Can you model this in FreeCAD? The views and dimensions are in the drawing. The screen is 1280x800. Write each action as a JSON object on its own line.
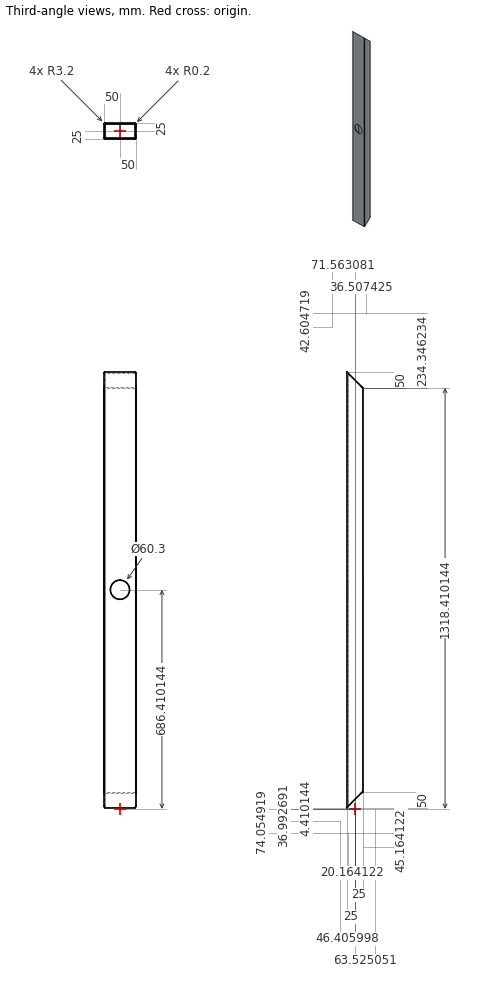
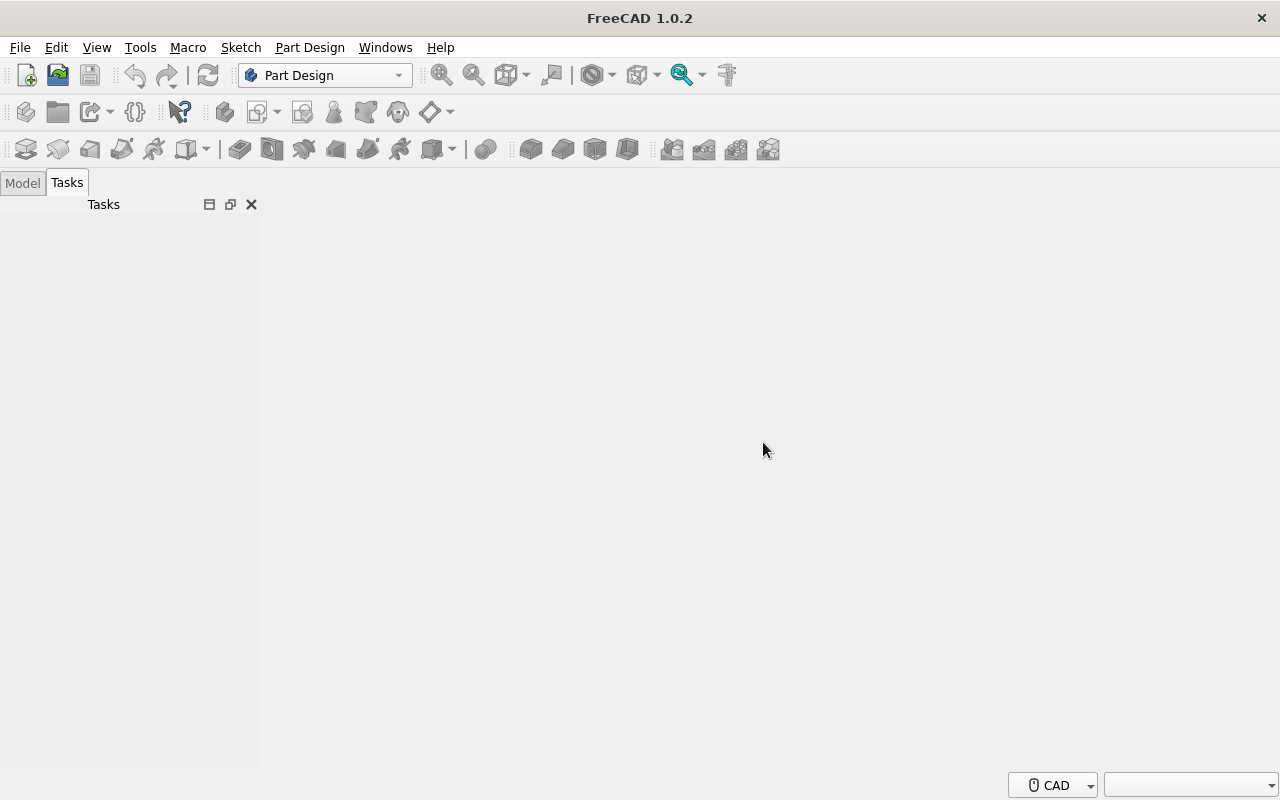
{"action": "left_click", "coordinate": [26, 76]}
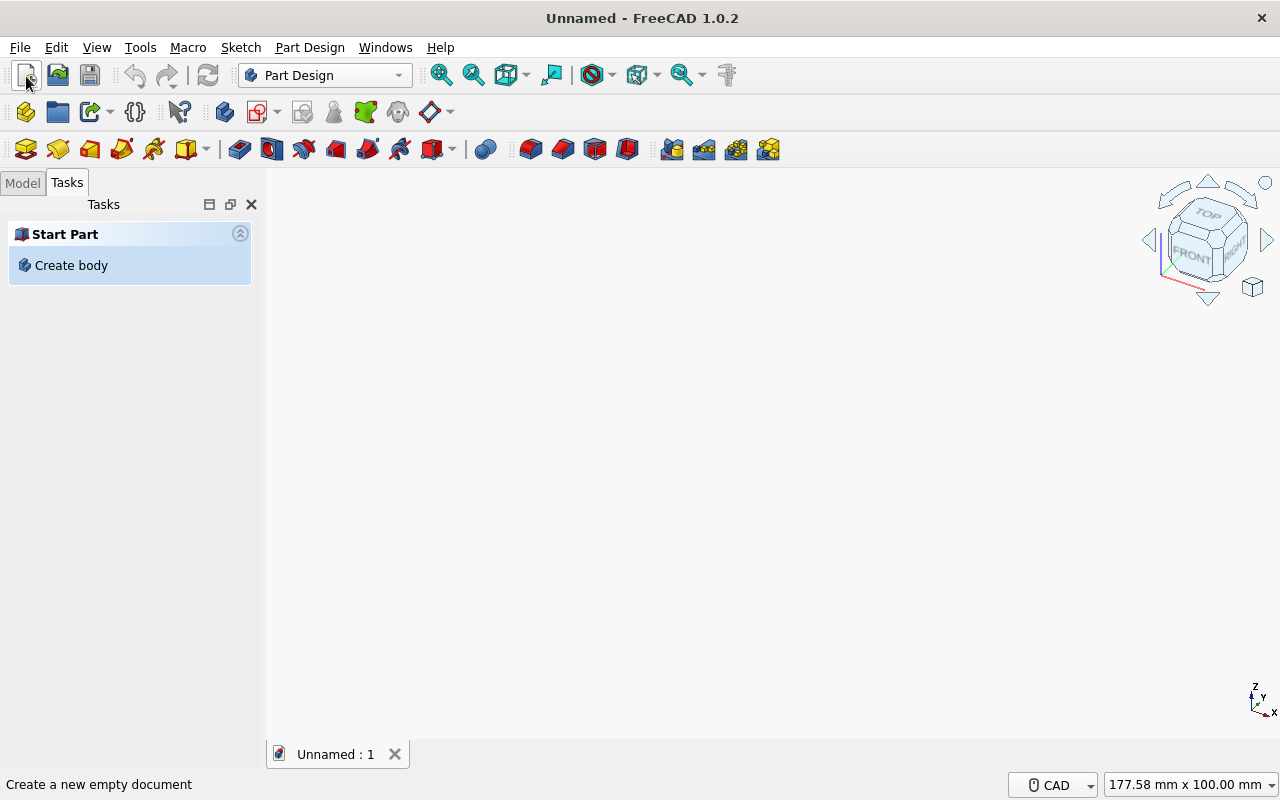
{"action": "left_click", "coordinate": [258, 112]}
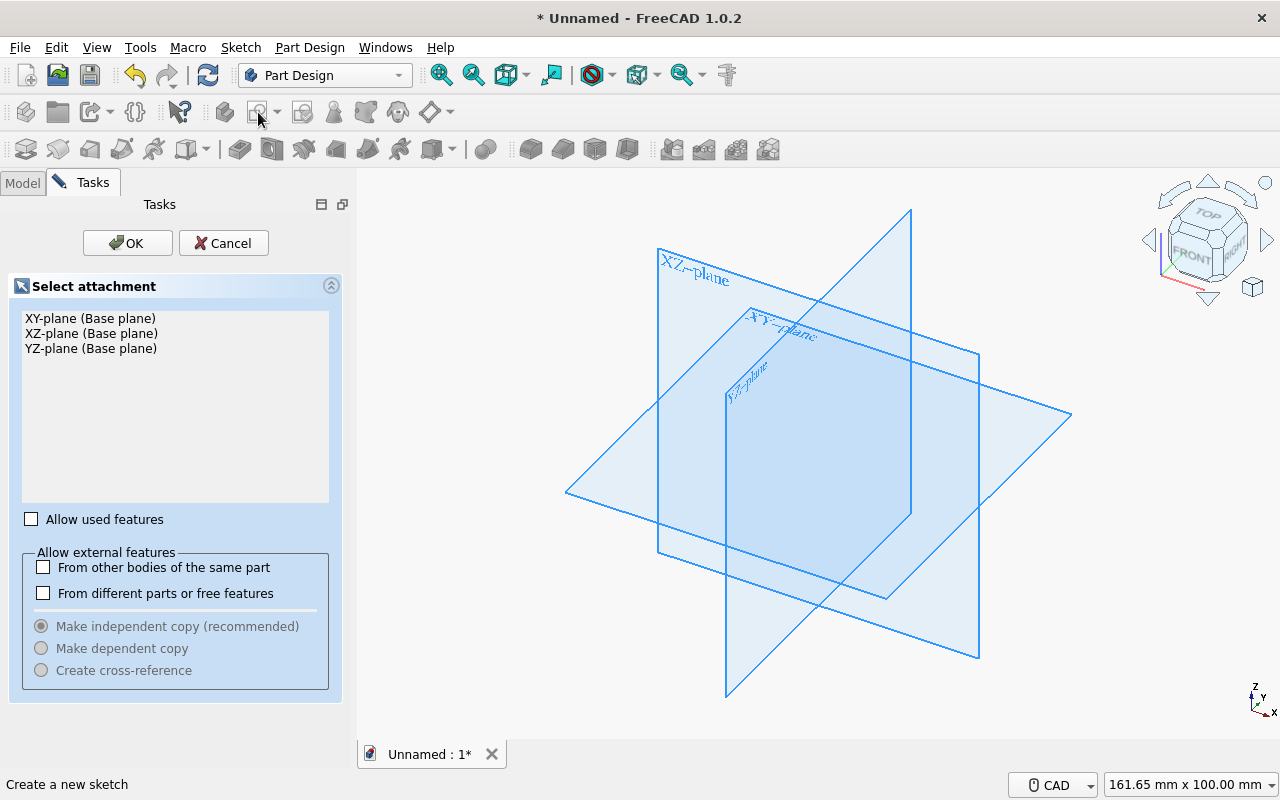
{"action": "left_click", "coordinate": [82, 318]}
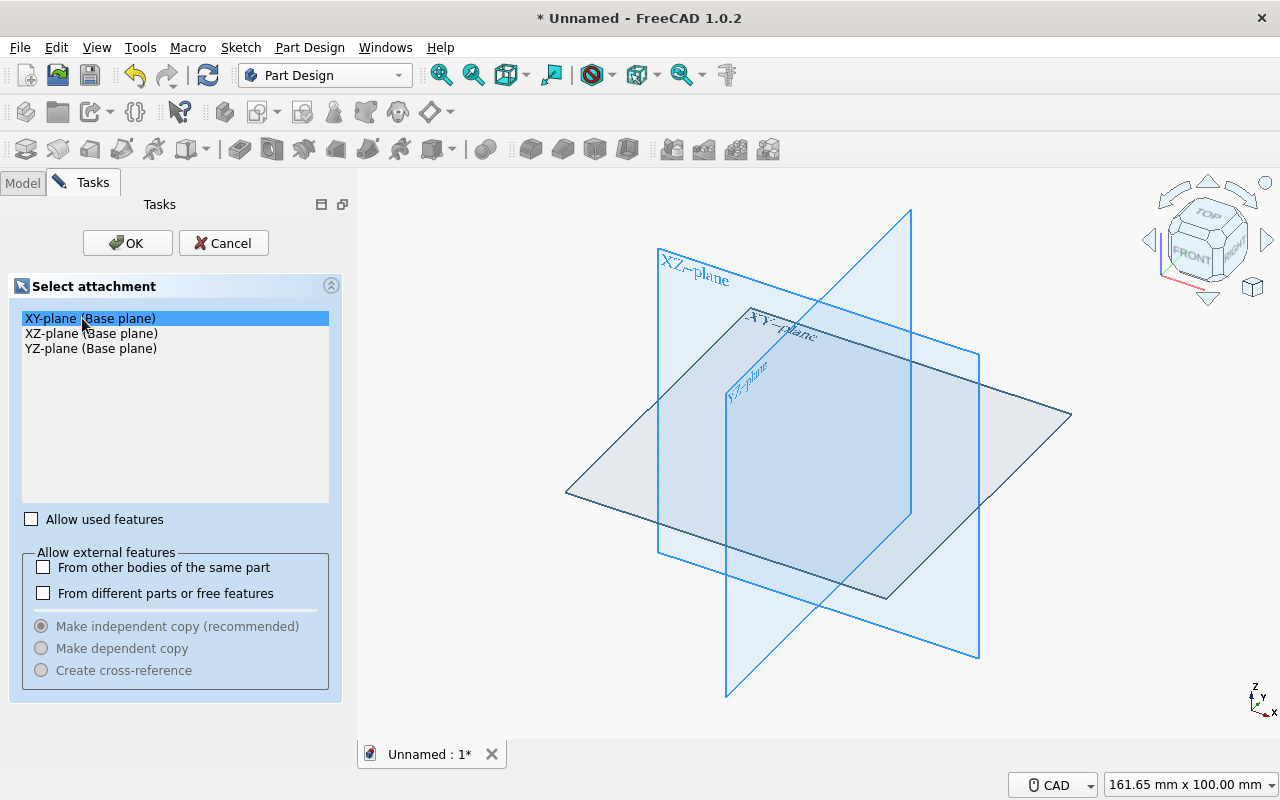
{"action": "left_click", "coordinate": [128, 243]}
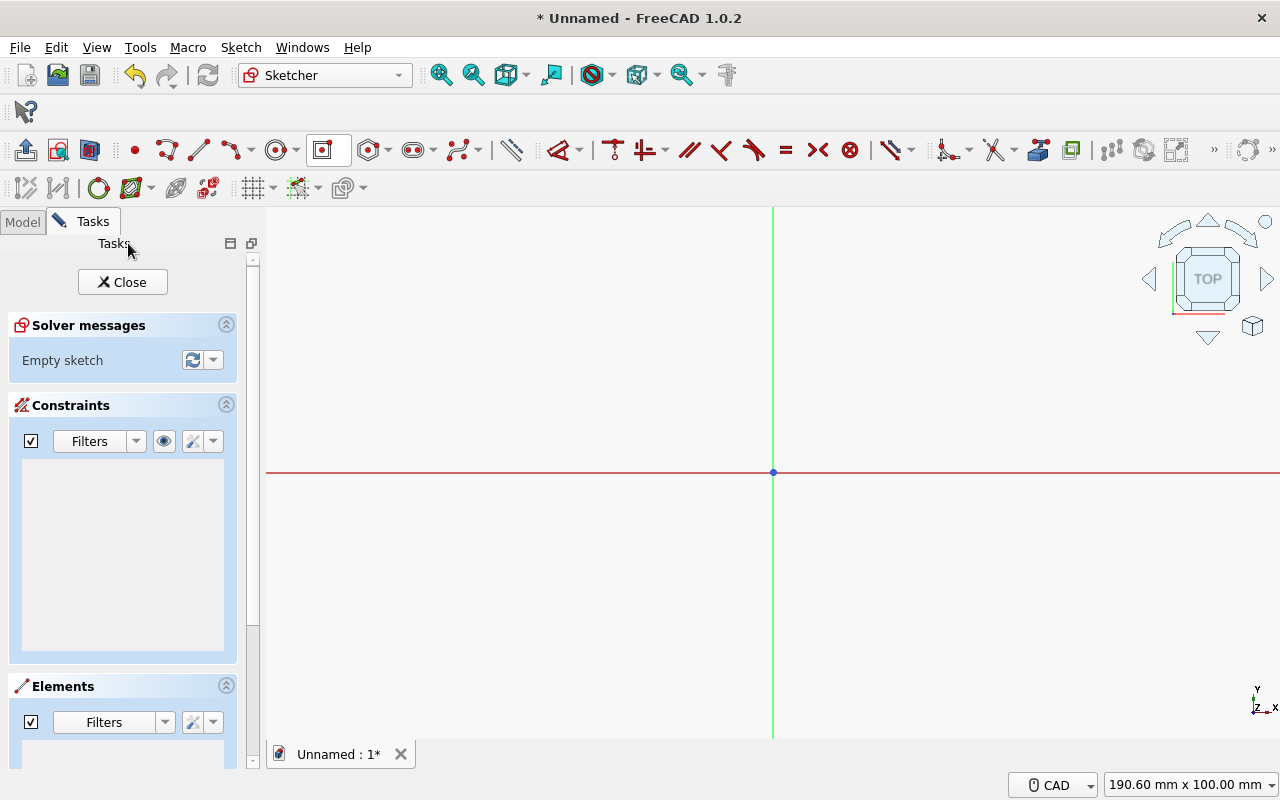
{"action": "left_click", "coordinate": [200, 150]}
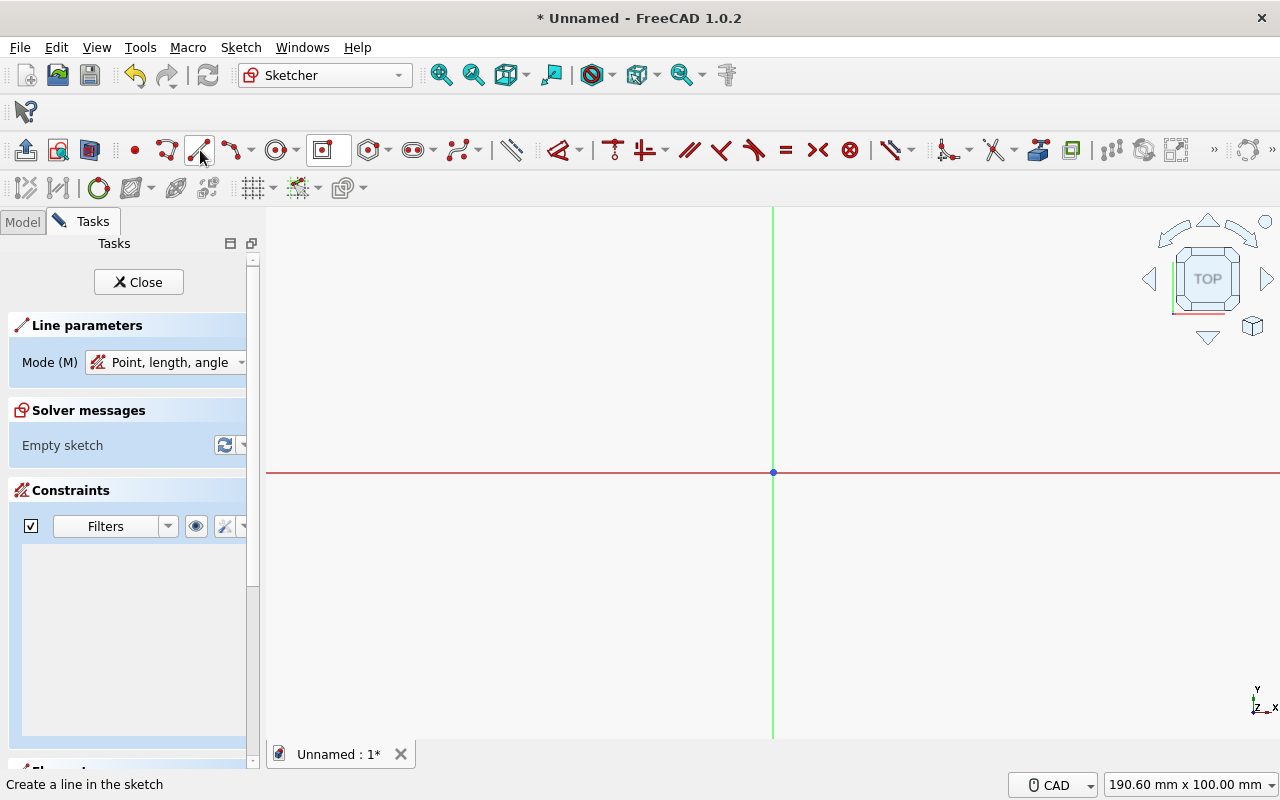
{"action": "left_click", "coordinate": [1022, 340]}
{"action": "left_click", "coordinate": [524, 340]}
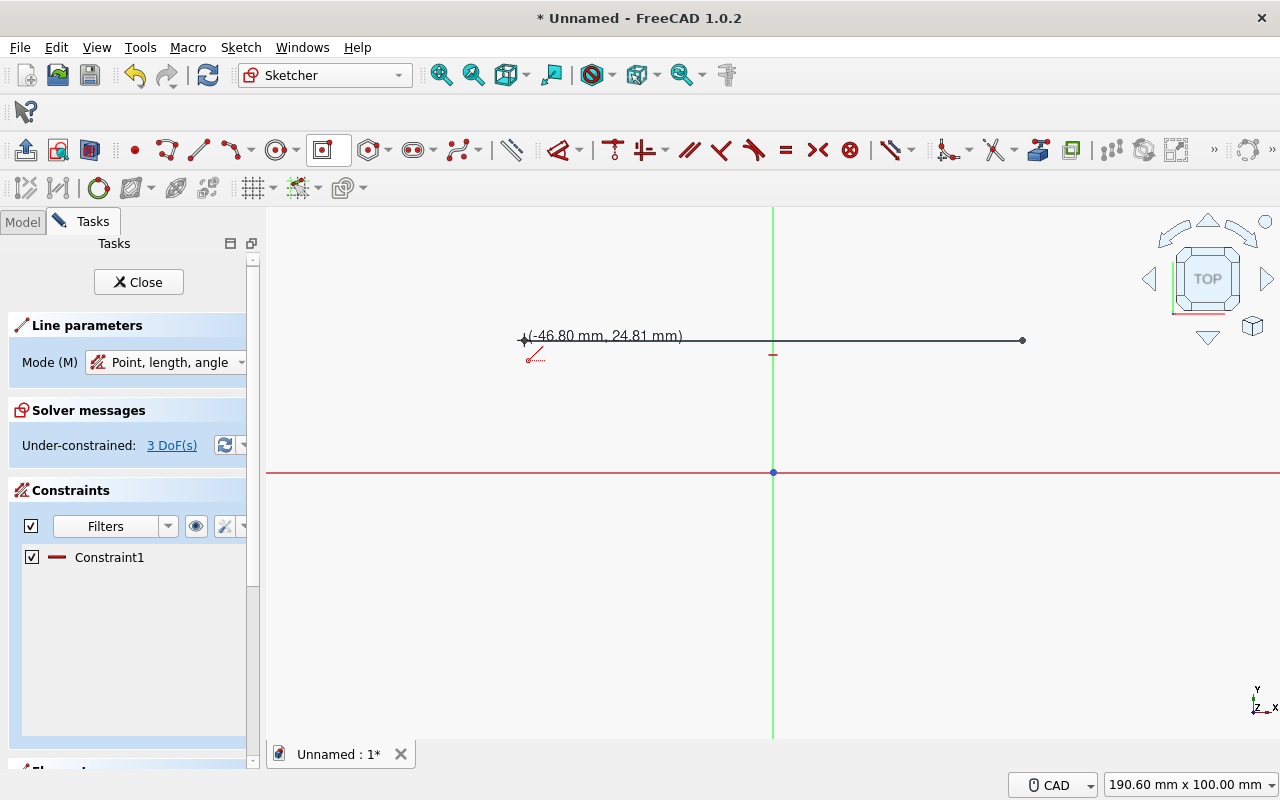
{"action": "left_click", "coordinate": [507, 357]}
{"action": "left_click", "coordinate": [507, 589]}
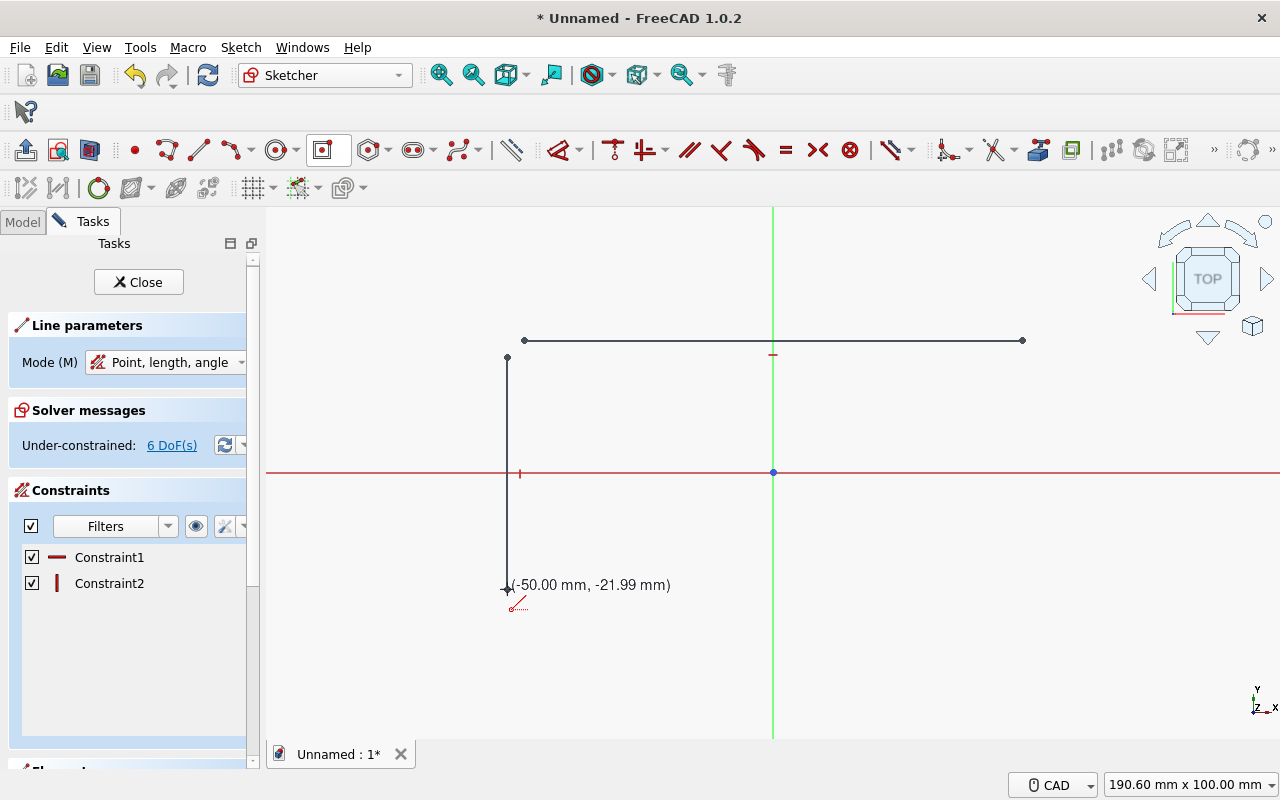
{"action": "left_click", "coordinate": [524, 606]}
{"action": "left_click", "coordinate": [1022, 606]}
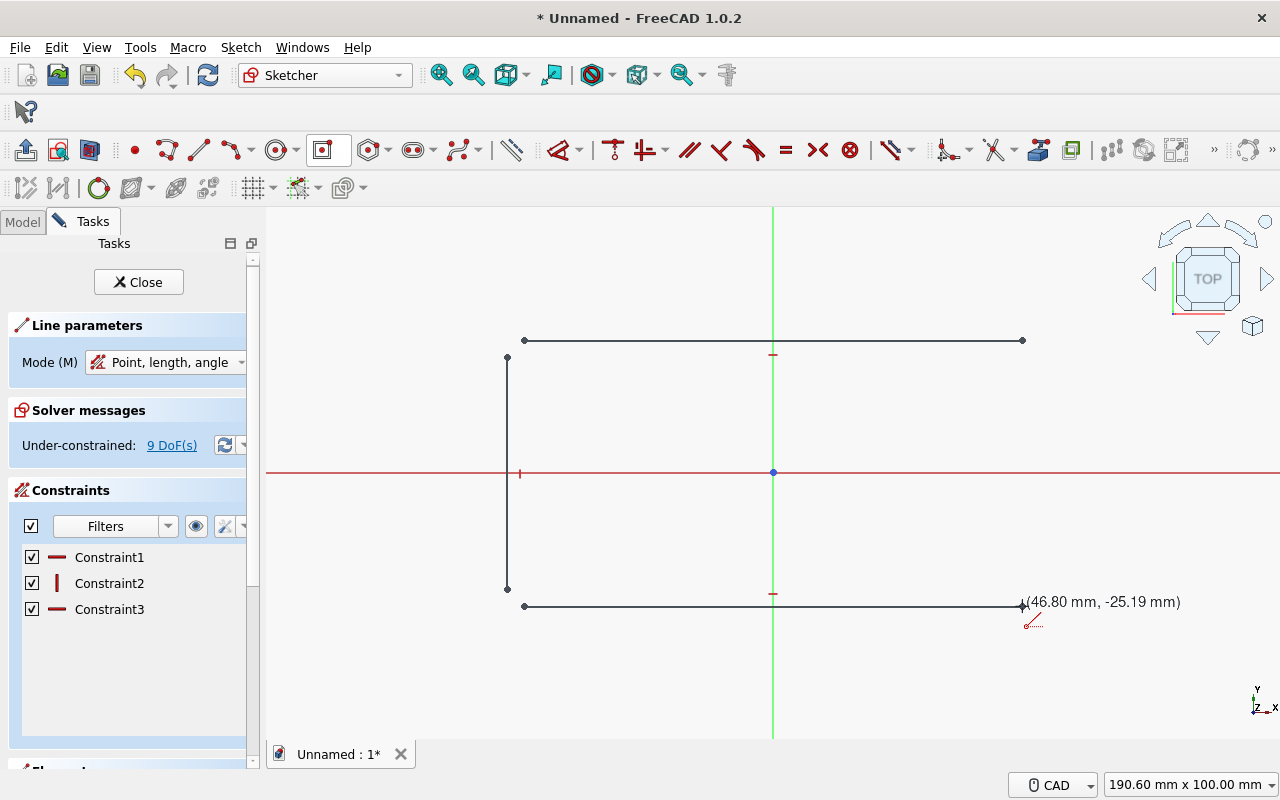
{"action": "left_click", "coordinate": [1039, 589]}
{"action": "left_click", "coordinate": [1039, 357]}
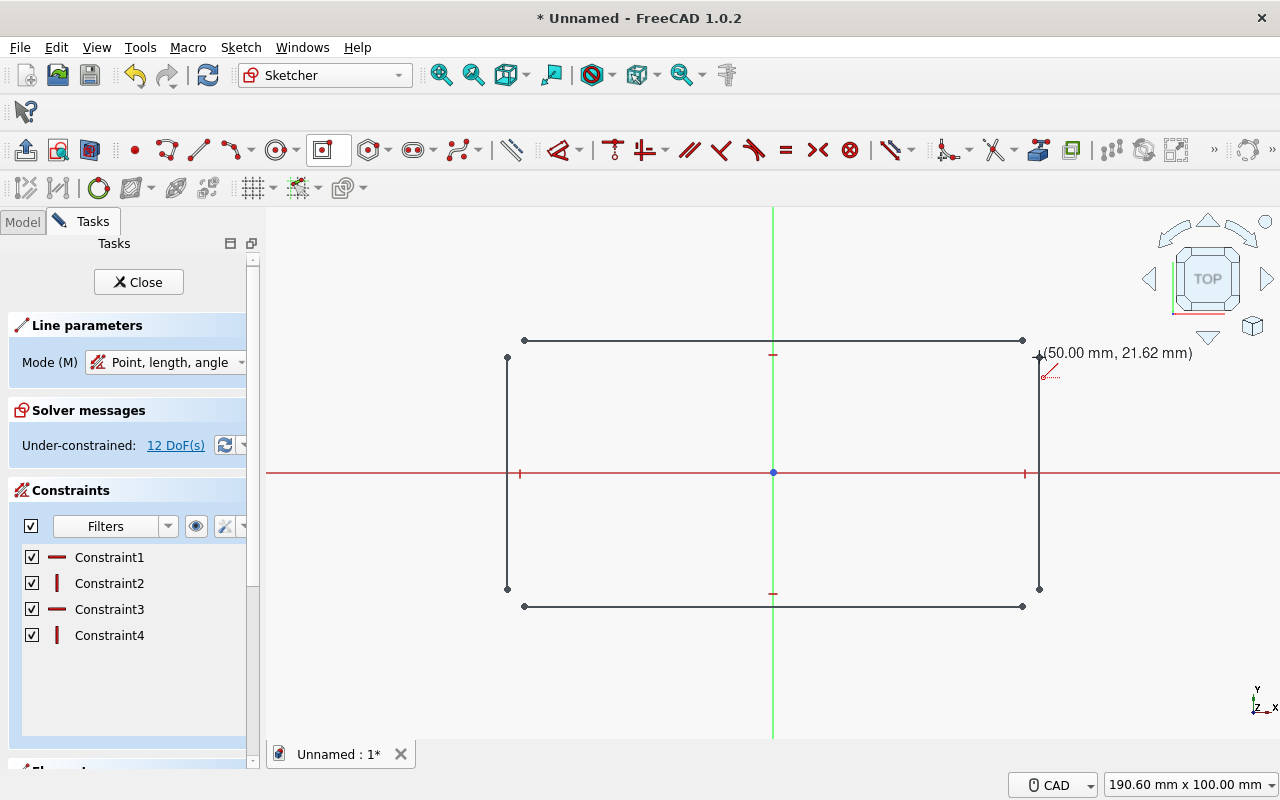
{"action": "left_click", "coordinate": [232, 150]}